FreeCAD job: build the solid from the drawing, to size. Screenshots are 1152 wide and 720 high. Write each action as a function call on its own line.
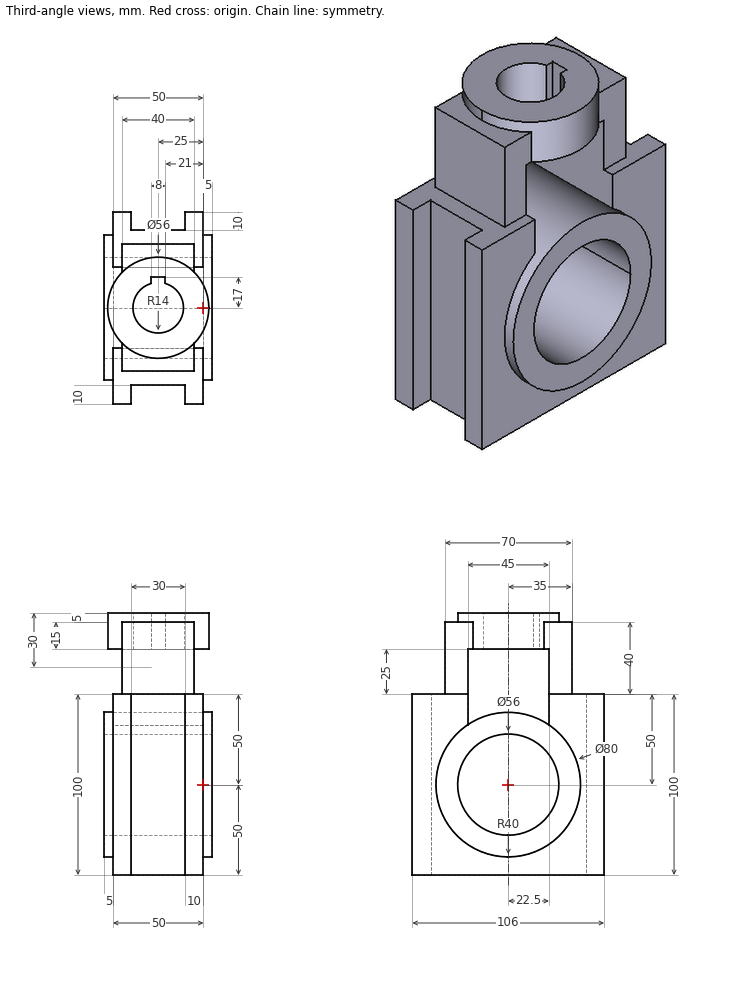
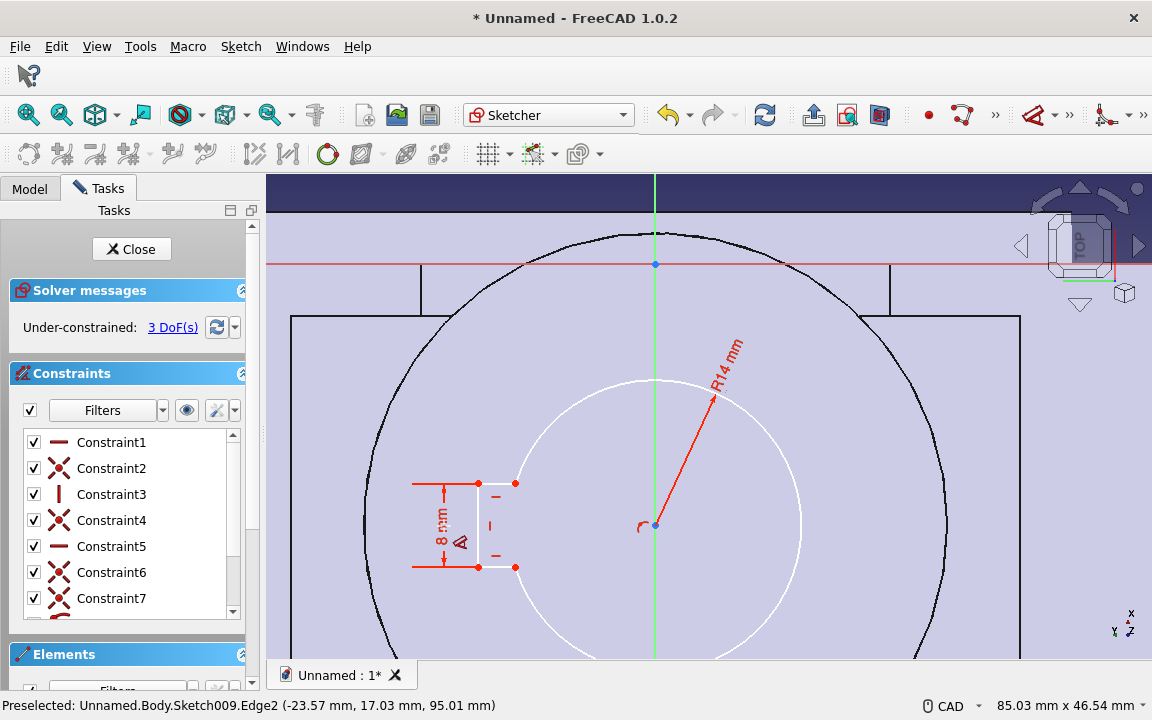
click(516, 484)
click(482, 374)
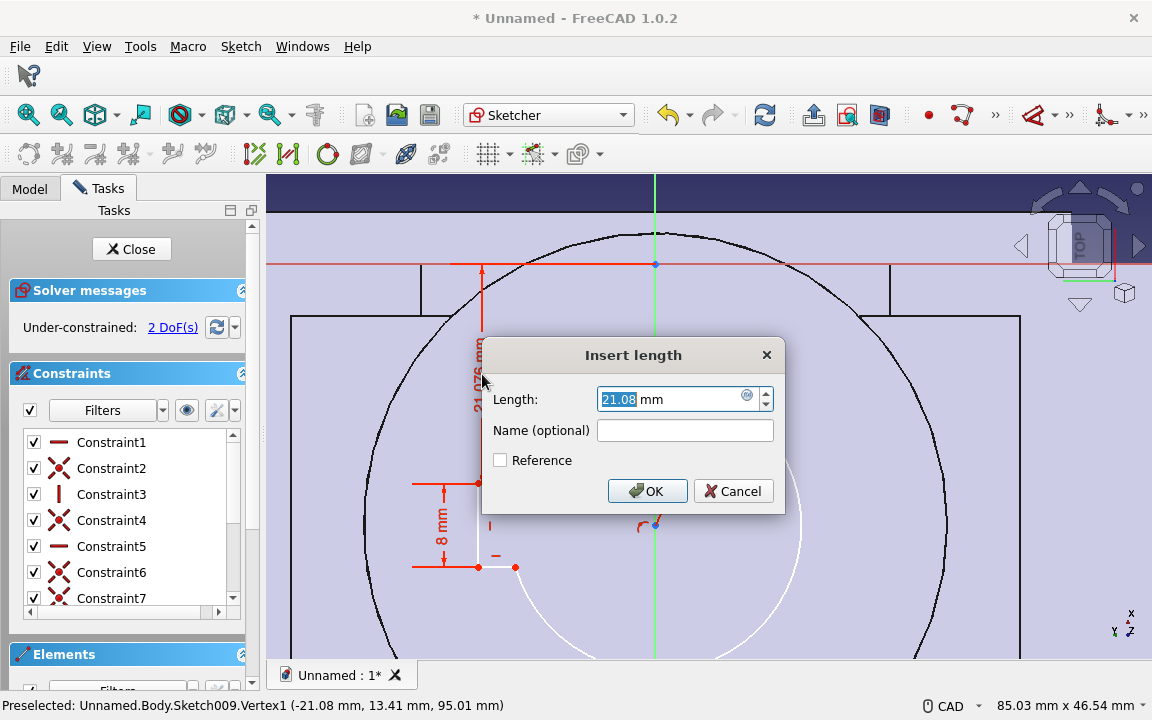
text(21)
key(Return)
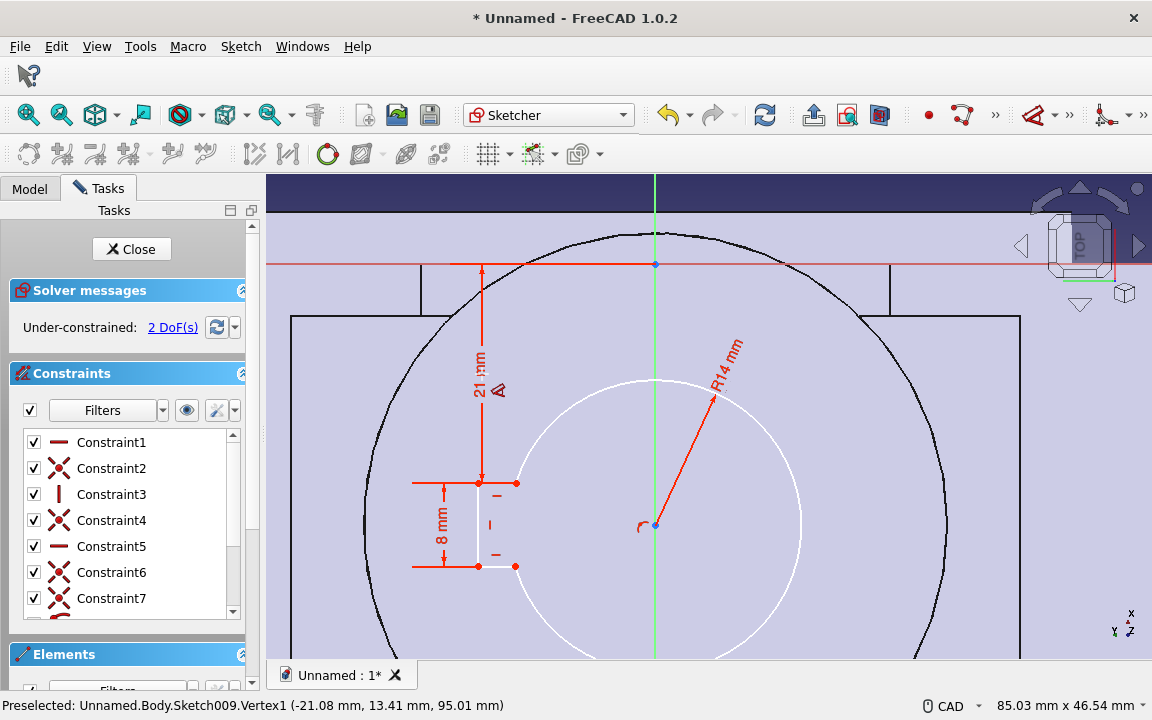
click(478, 483)
click(567, 230)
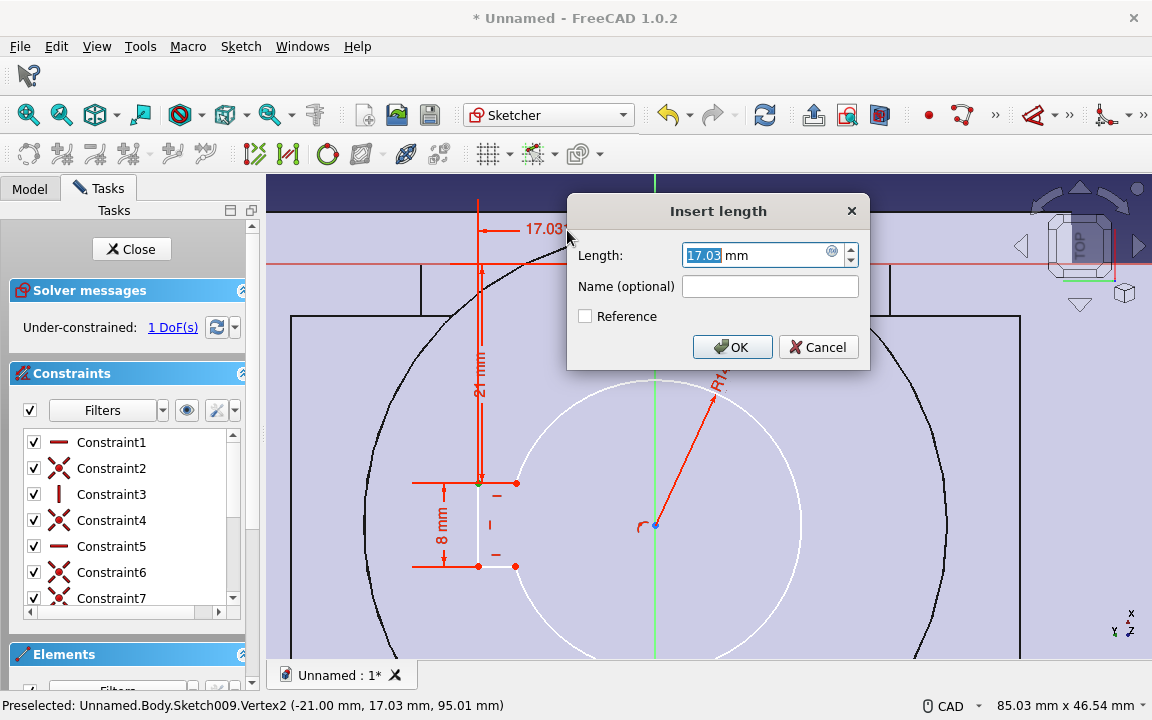
text(17)
key(Return)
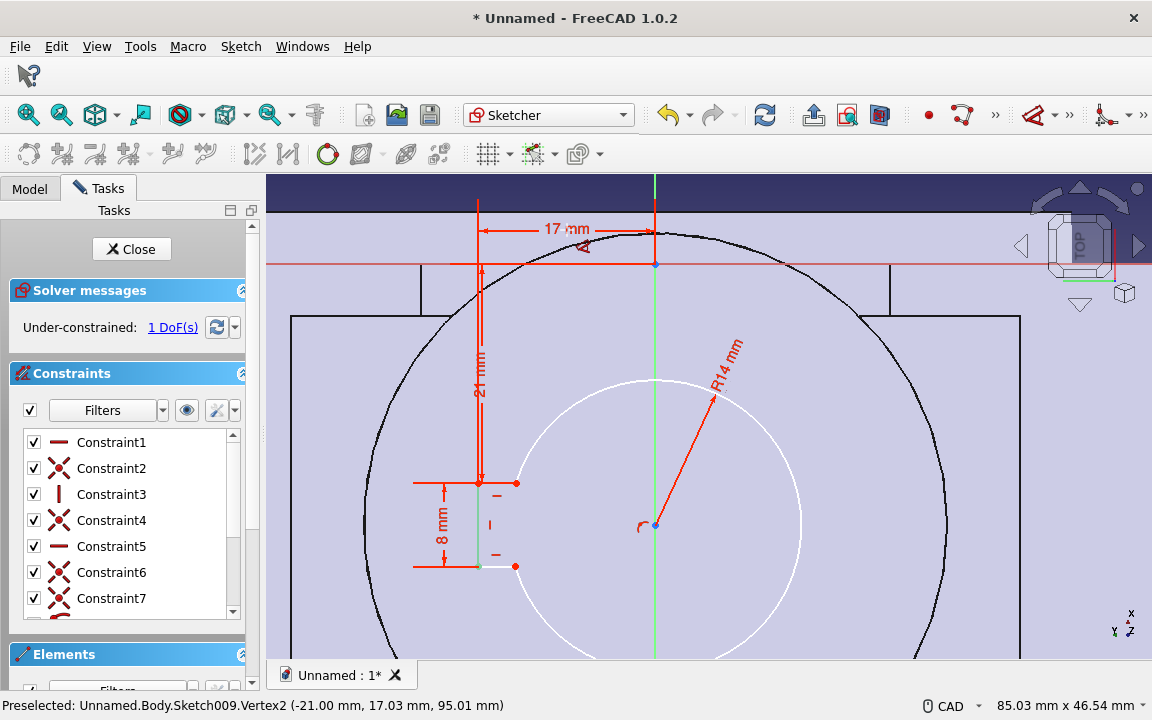
click(655, 526)
click(689, 335)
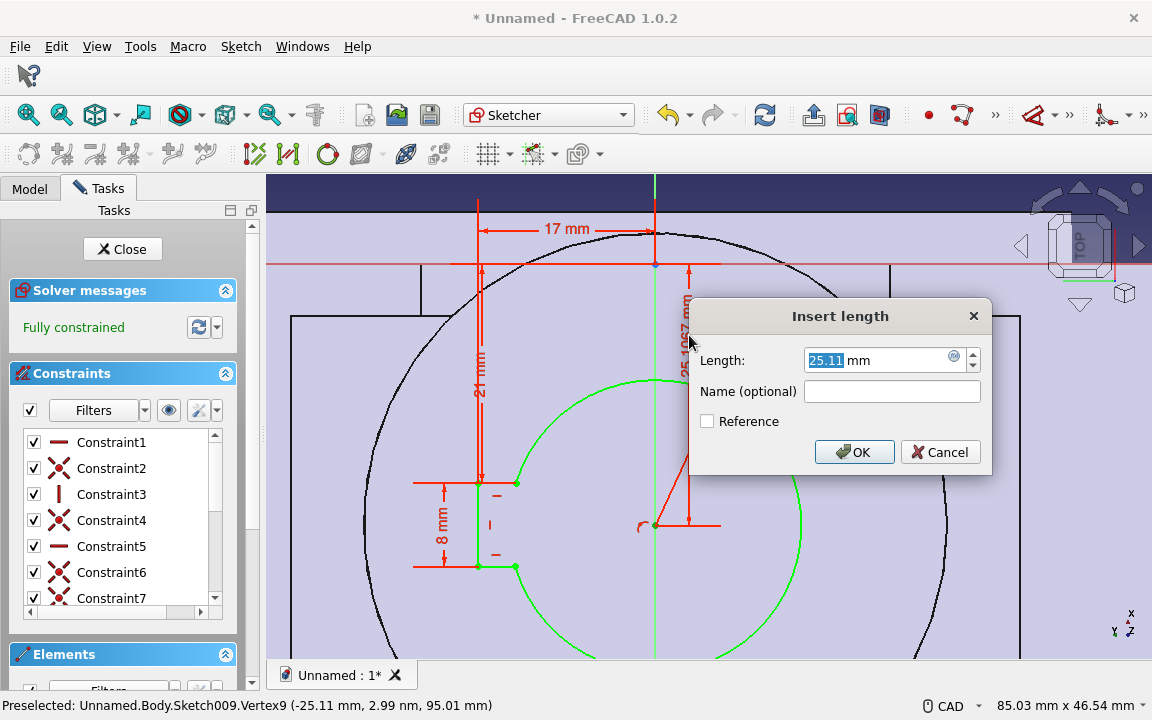
text(25)
key(Return)
key(Escape)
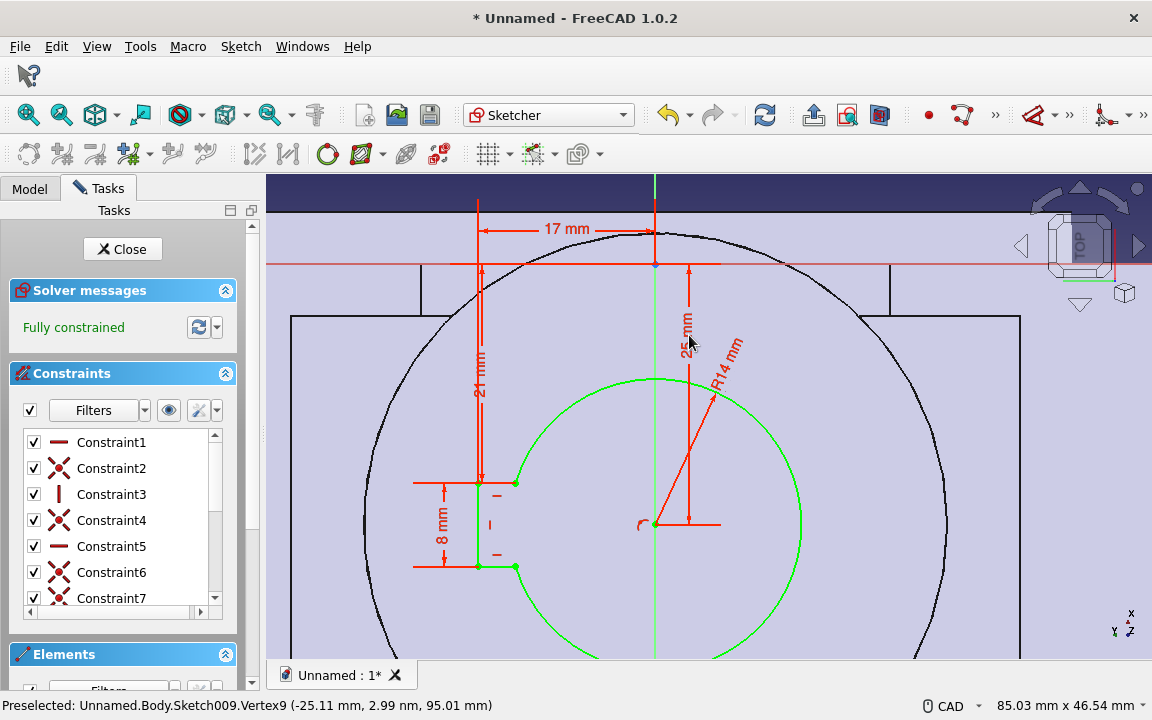
click(123, 249)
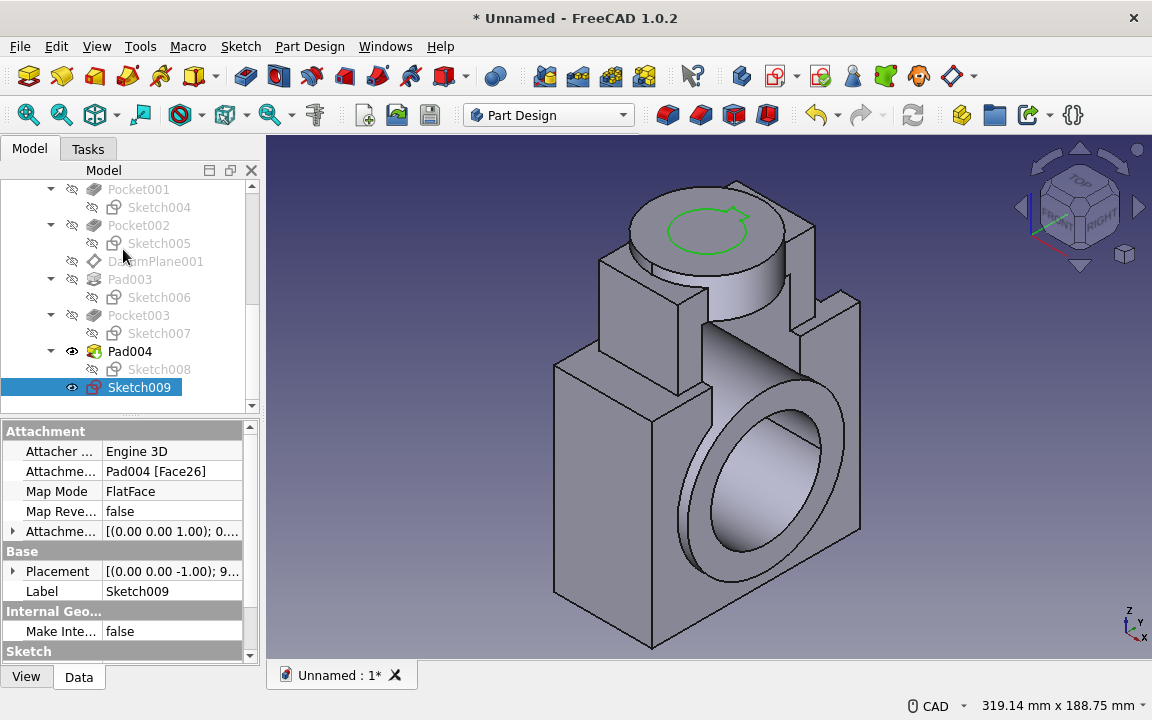
click(246, 76)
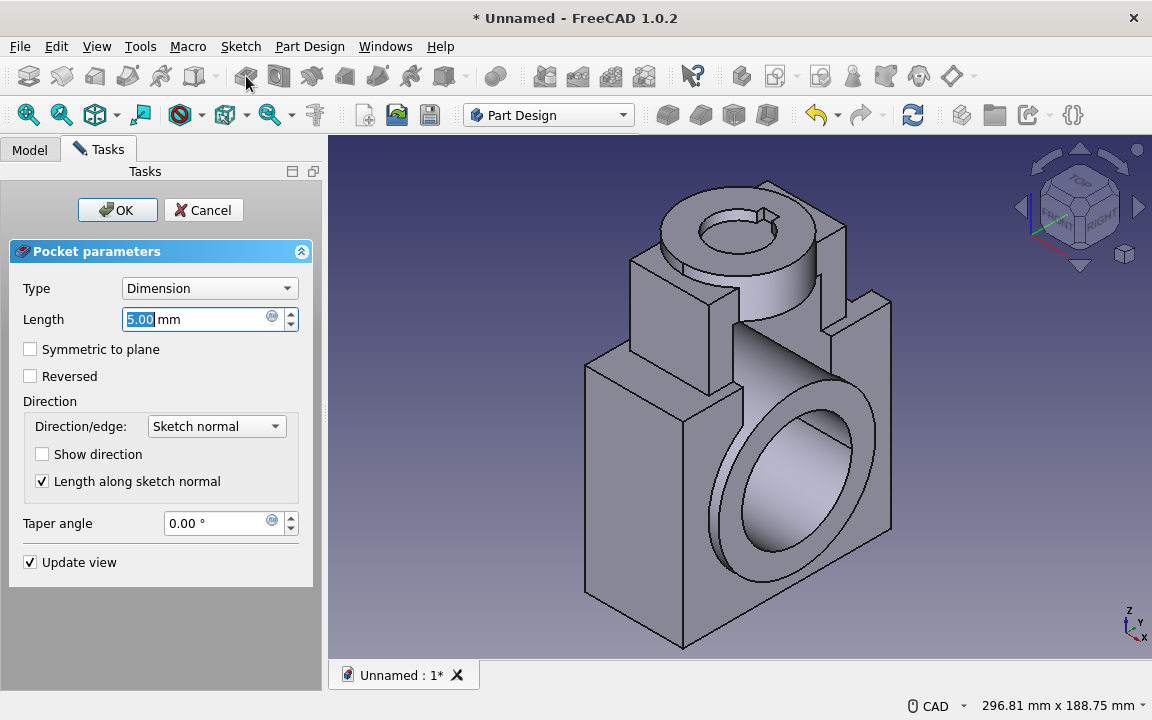
text(30)
key(Tab)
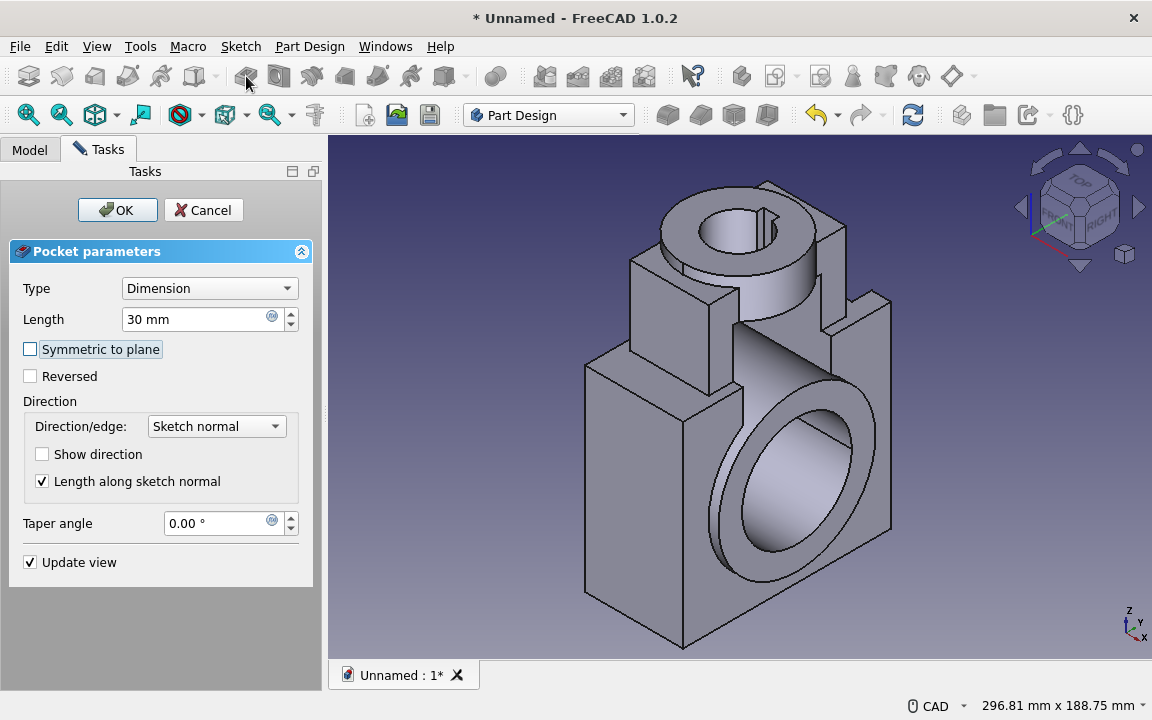
click(118, 210)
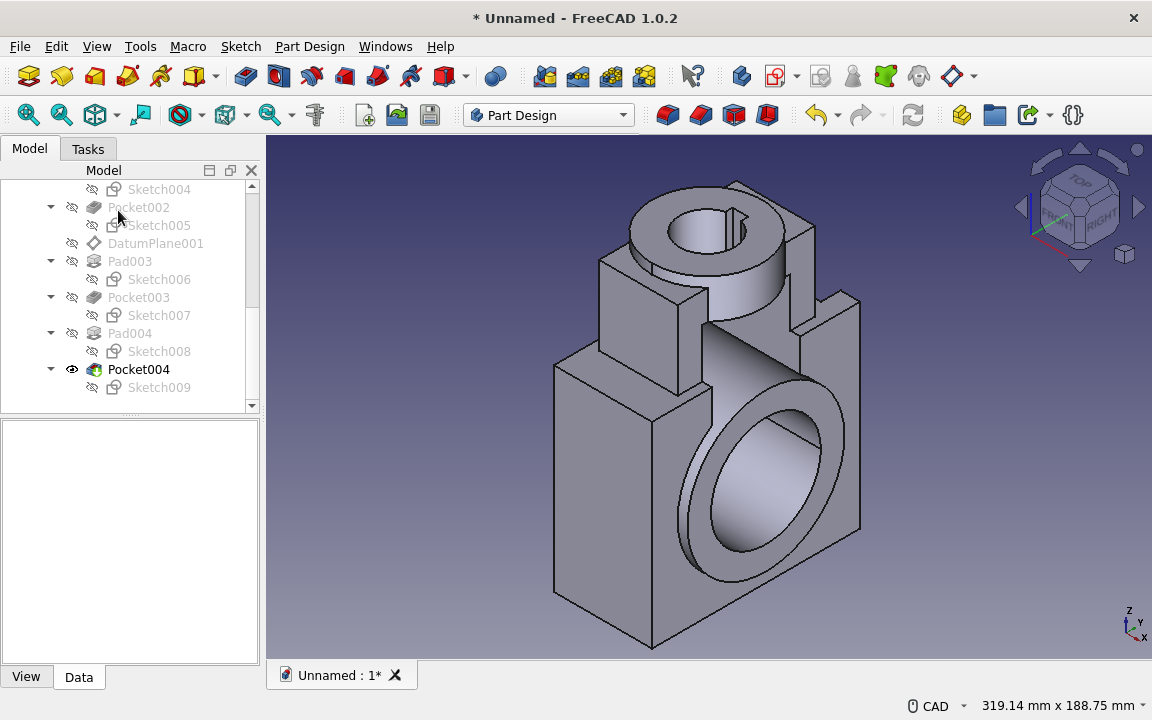
key(6)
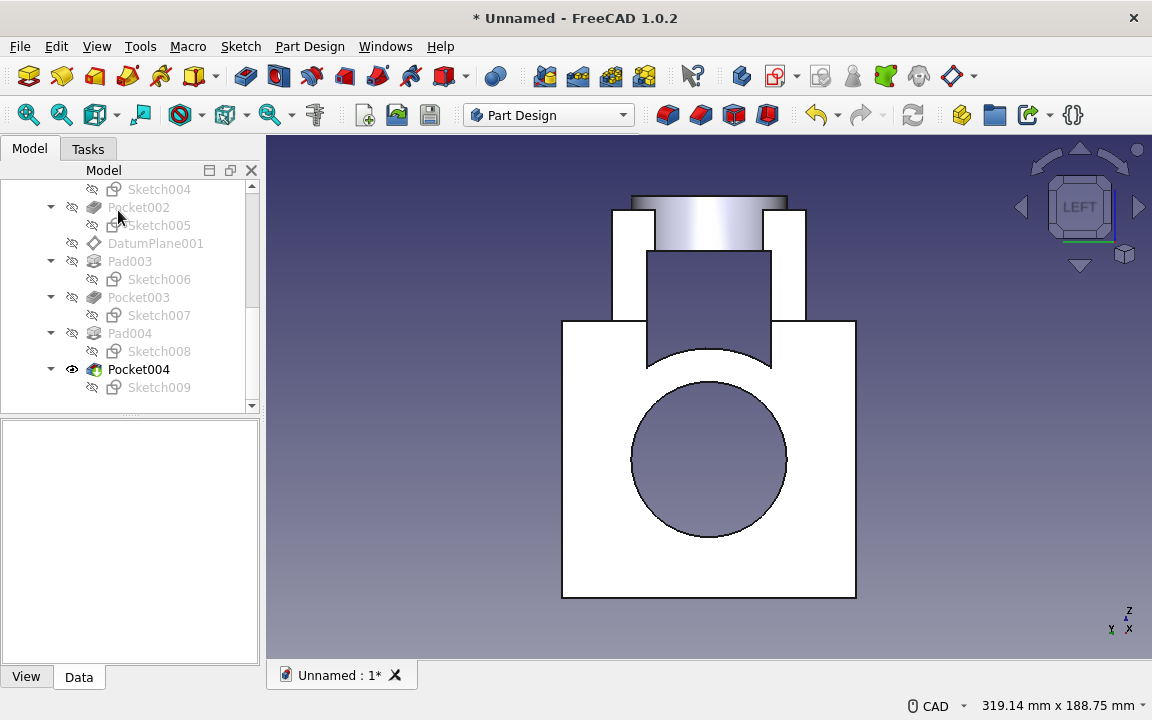
click(625, 538)